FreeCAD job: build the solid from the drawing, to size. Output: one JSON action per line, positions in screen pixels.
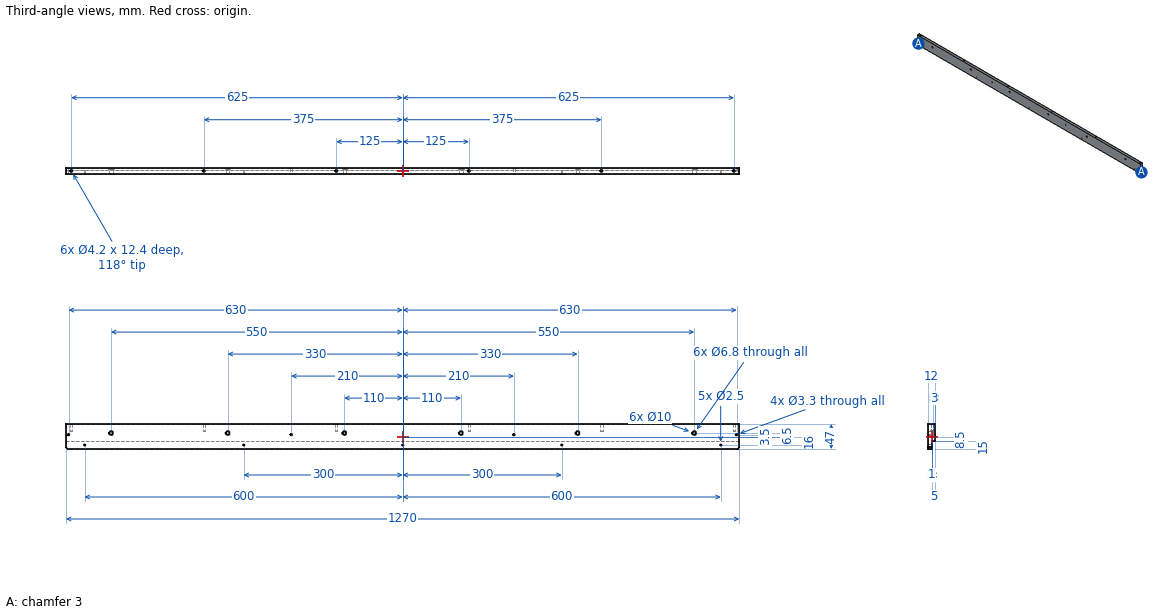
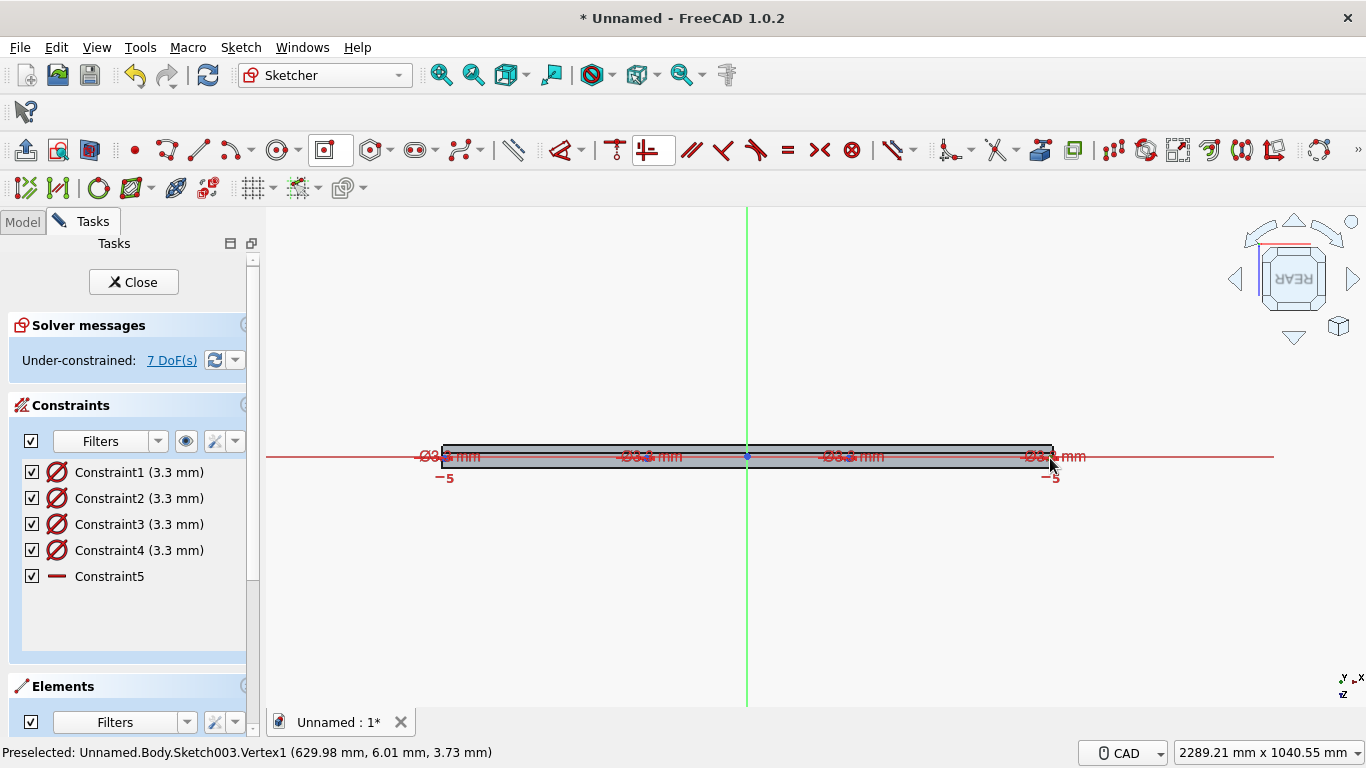
{"action": "left_click", "coordinate": [848, 458]}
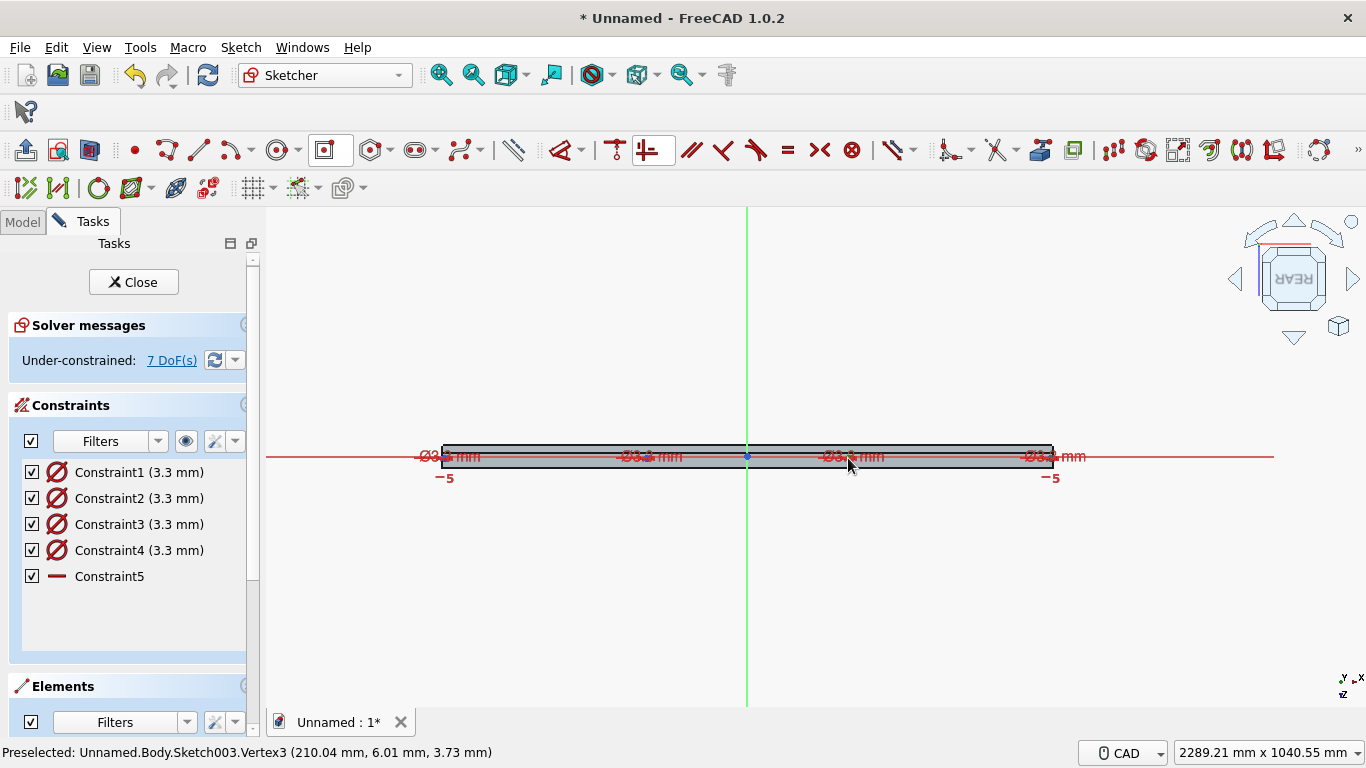
{"action": "key", "text": "h"}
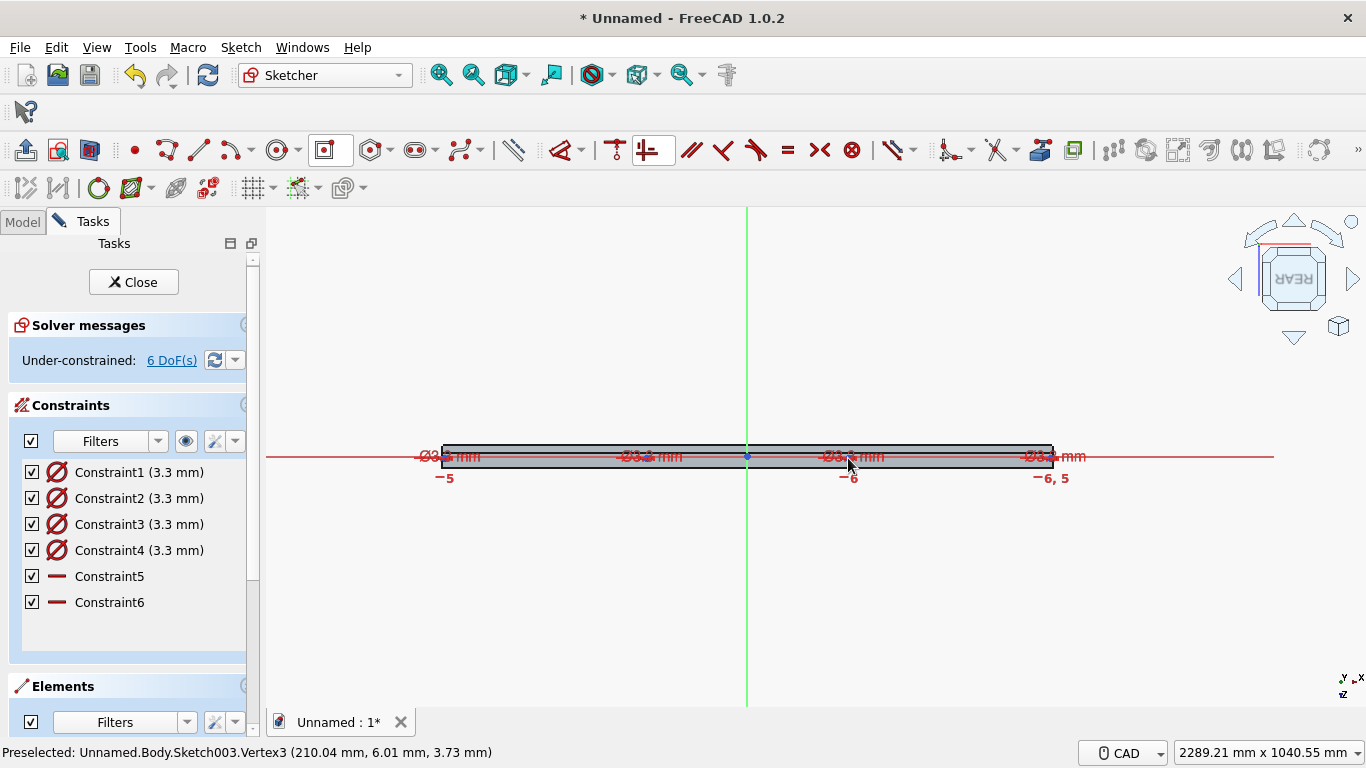
{"action": "left_click", "coordinate": [445, 458]}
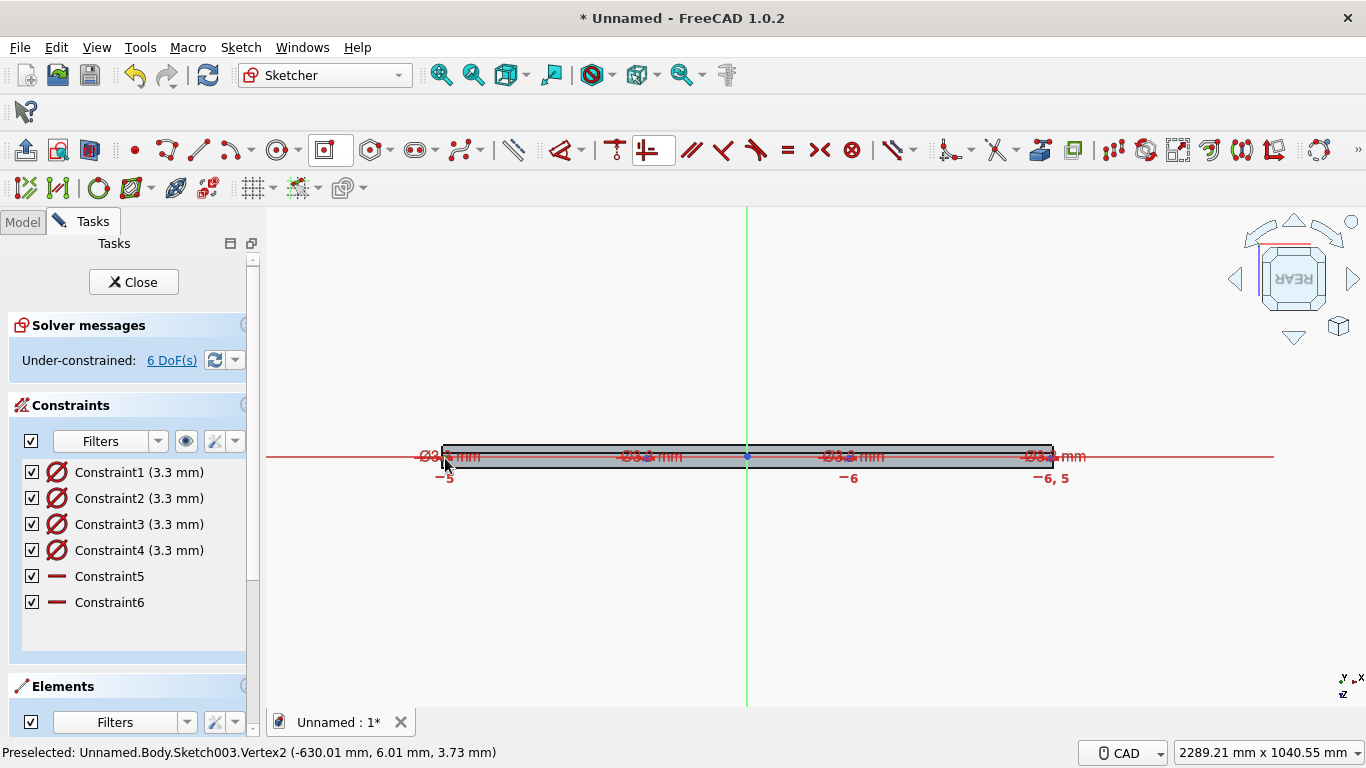
{"action": "left_click", "coordinate": [647, 458]}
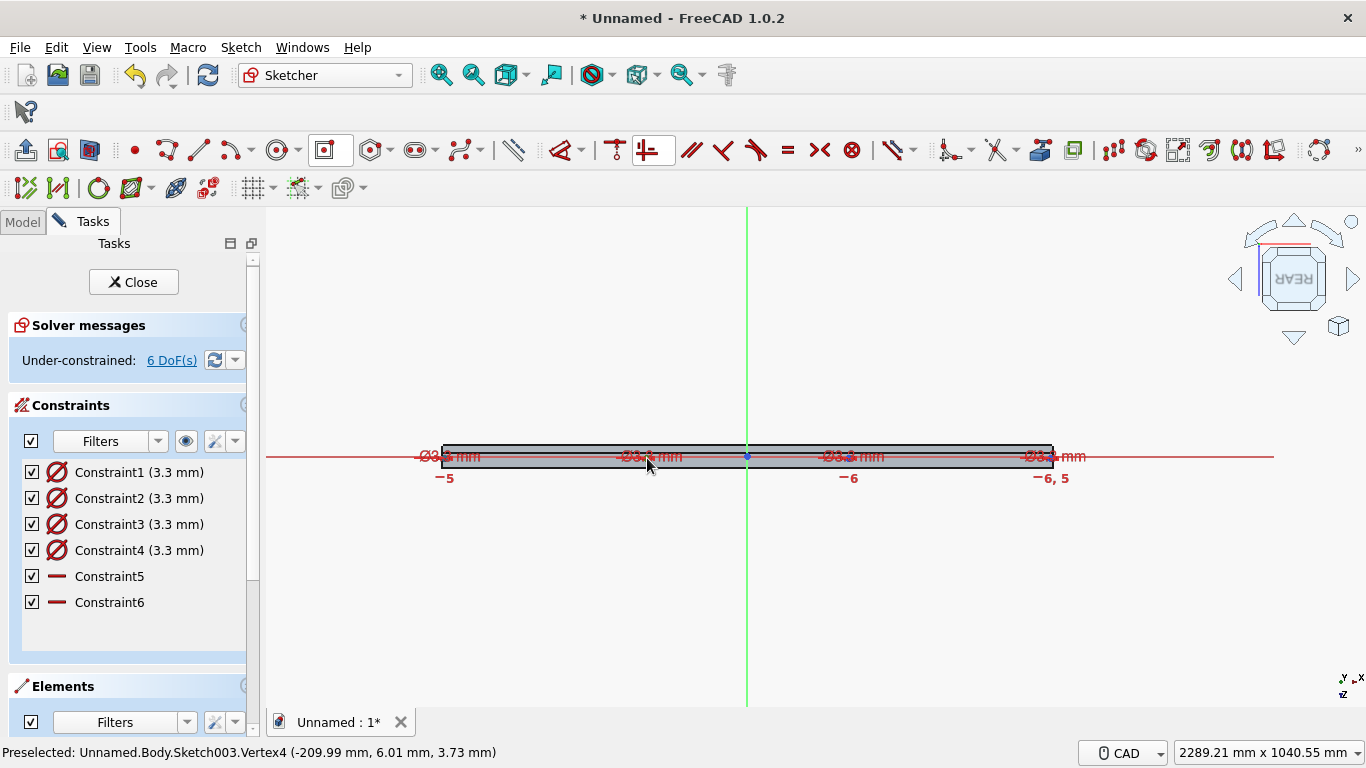
{"action": "key", "text": "h"}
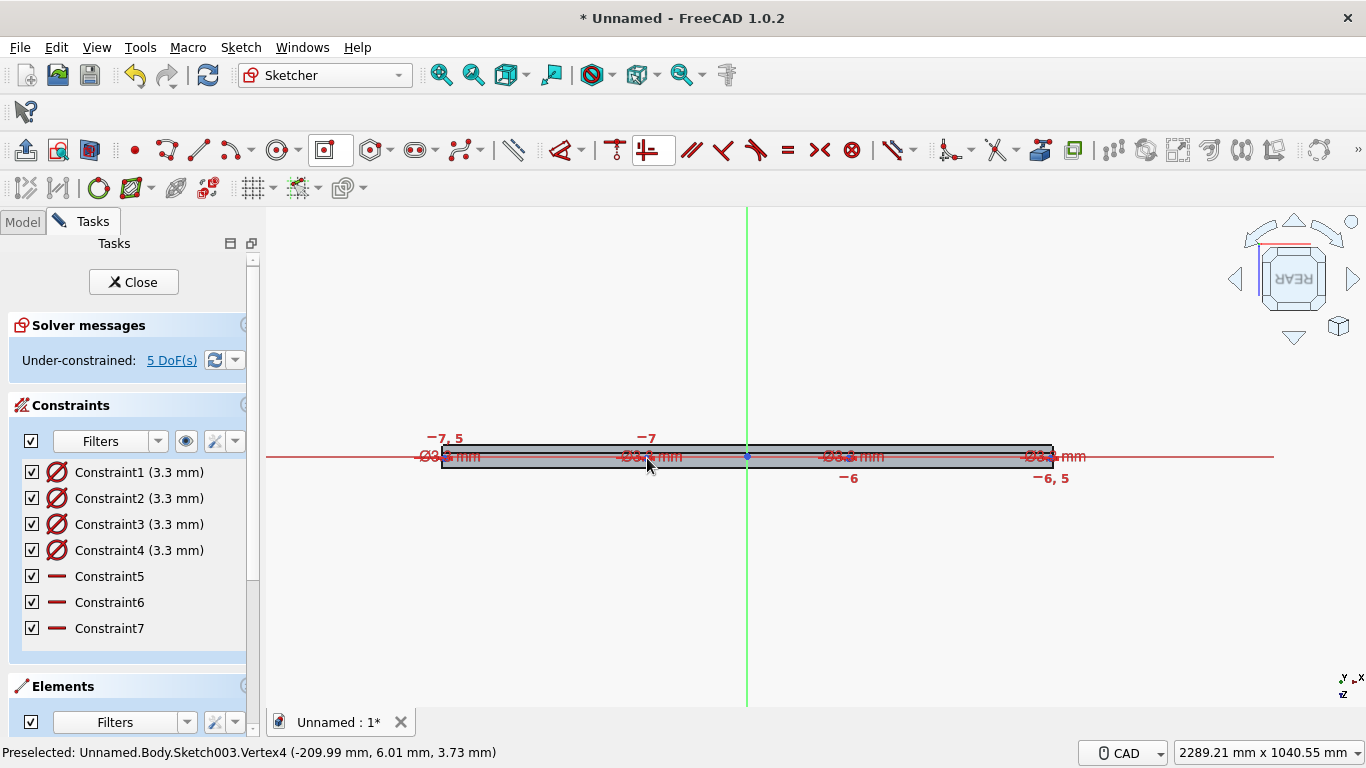
{"action": "left_click", "coordinate": [560, 150]}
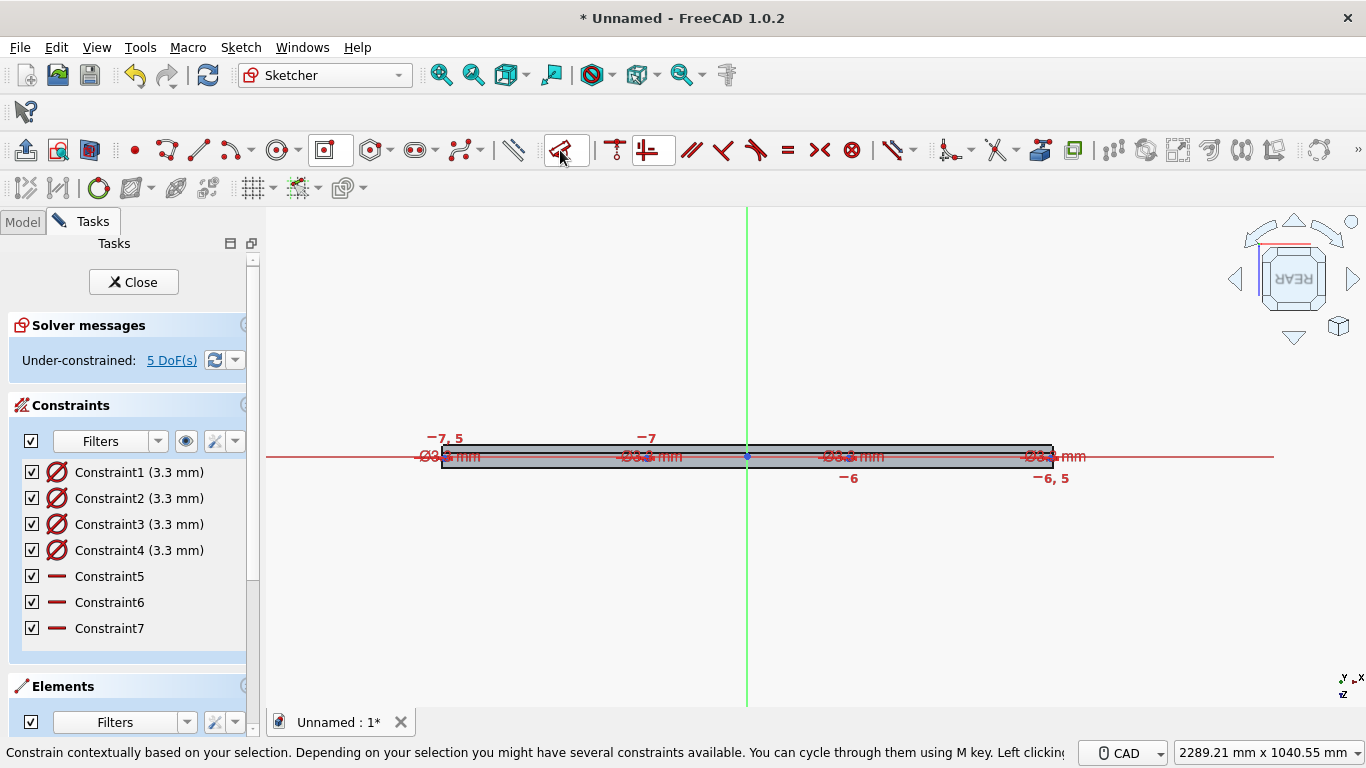
{"action": "left_click", "coordinate": [1050, 458]}
{"action": "left_click", "coordinate": [899, 423]}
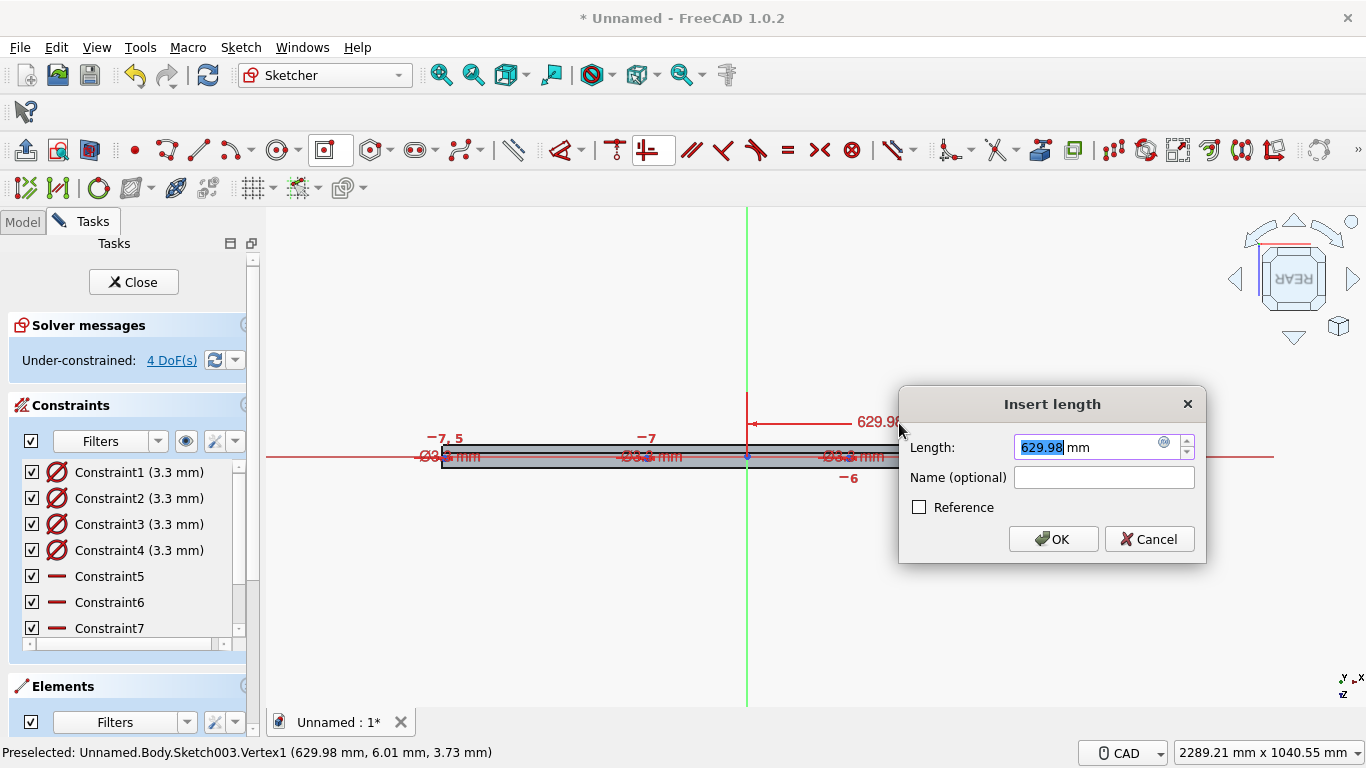
{"action": "type", "text": "630"}
{"action": "key", "text": "Return"}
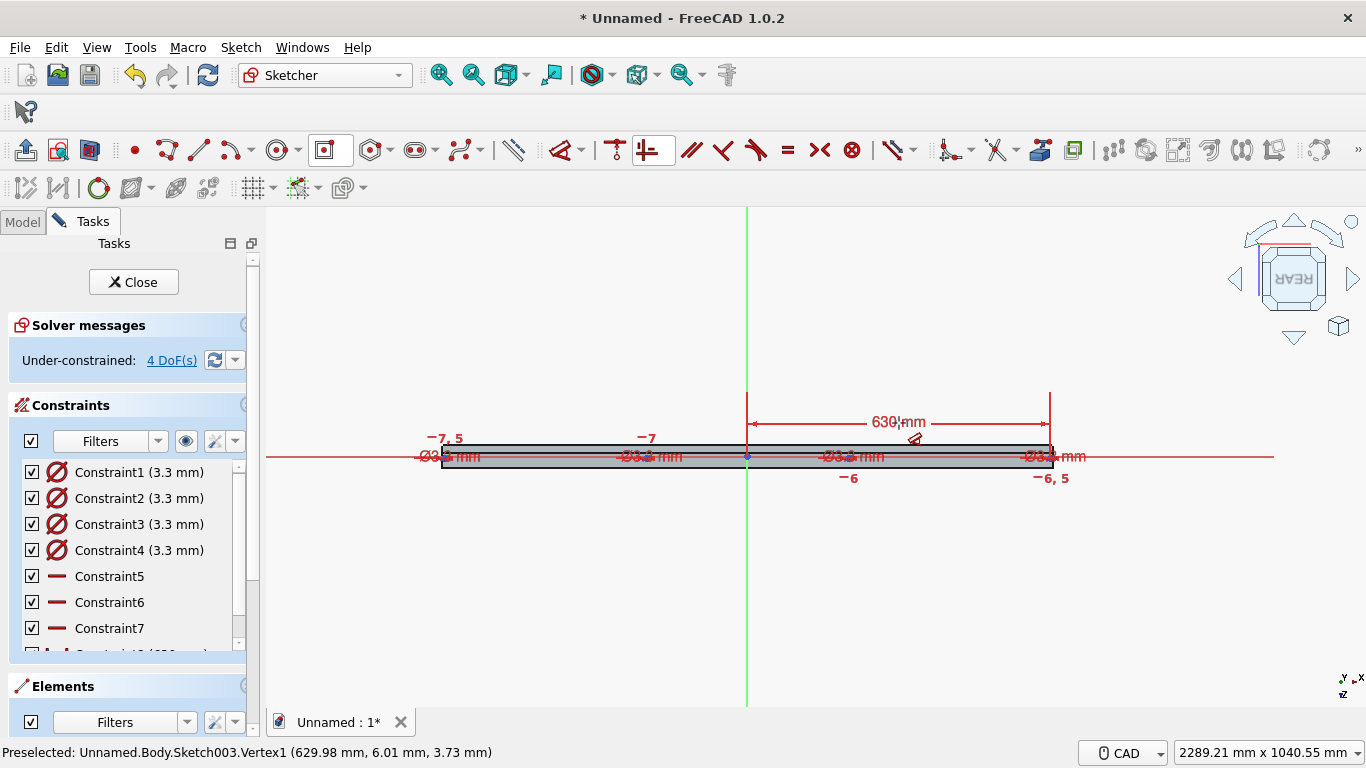
{"action": "scroll", "coordinate": [1050, 458], "scroll_direction": "up", "scroll_amount": 16}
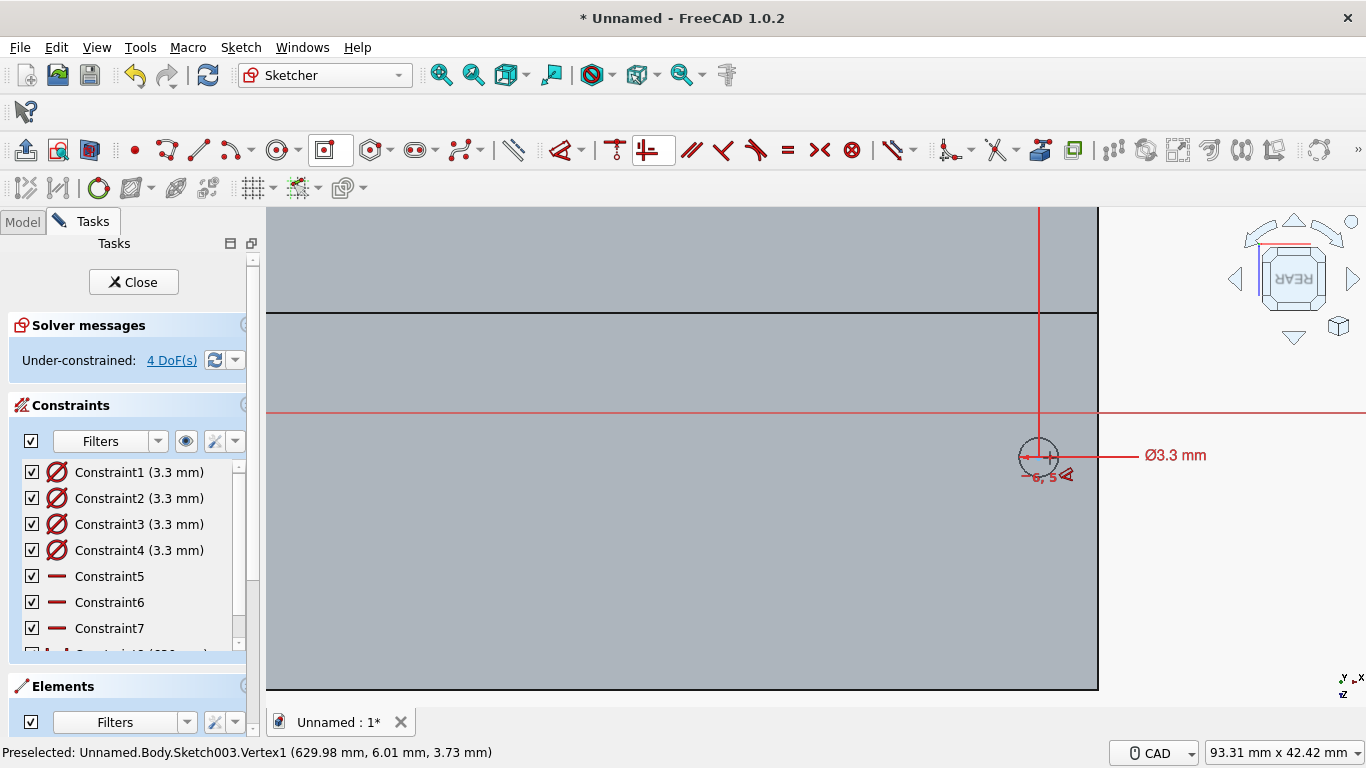
{"action": "left_click", "coordinate": [1039, 457]}
{"action": "left_click", "coordinate": [1073, 435]}